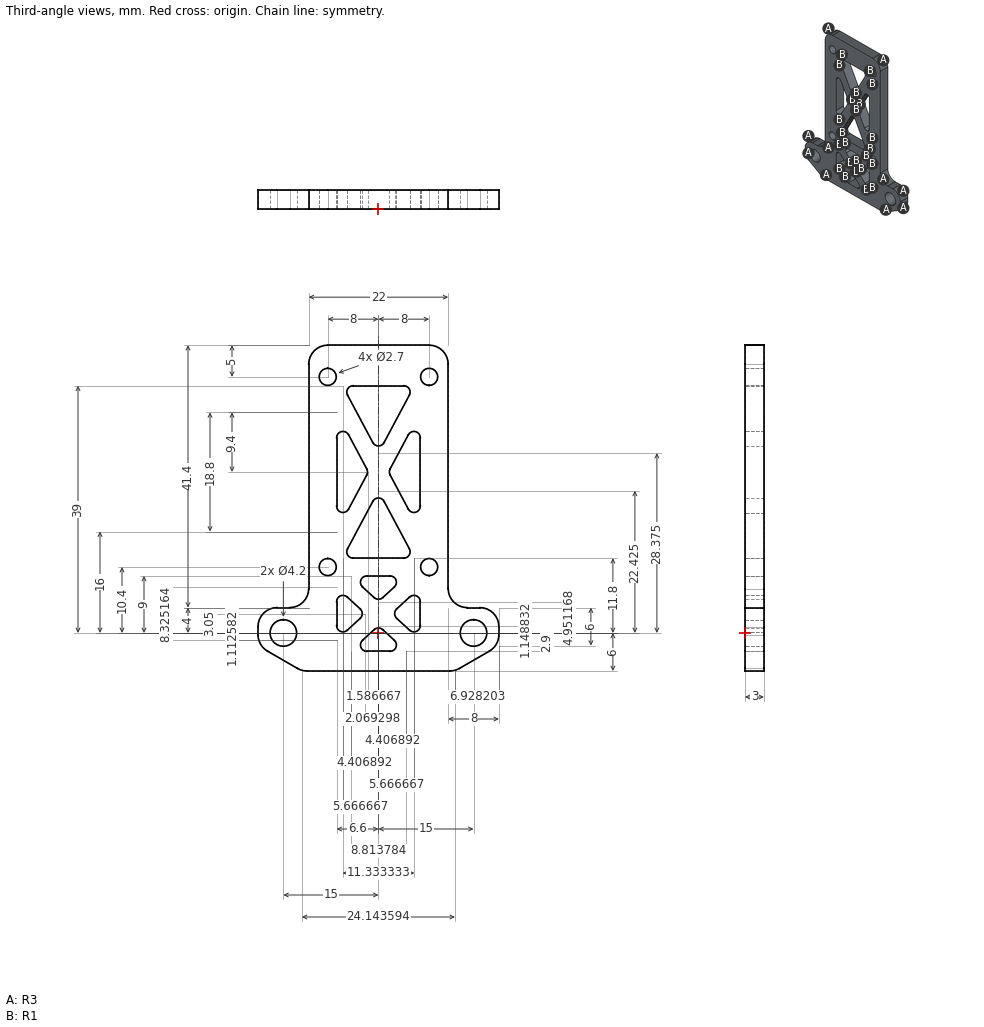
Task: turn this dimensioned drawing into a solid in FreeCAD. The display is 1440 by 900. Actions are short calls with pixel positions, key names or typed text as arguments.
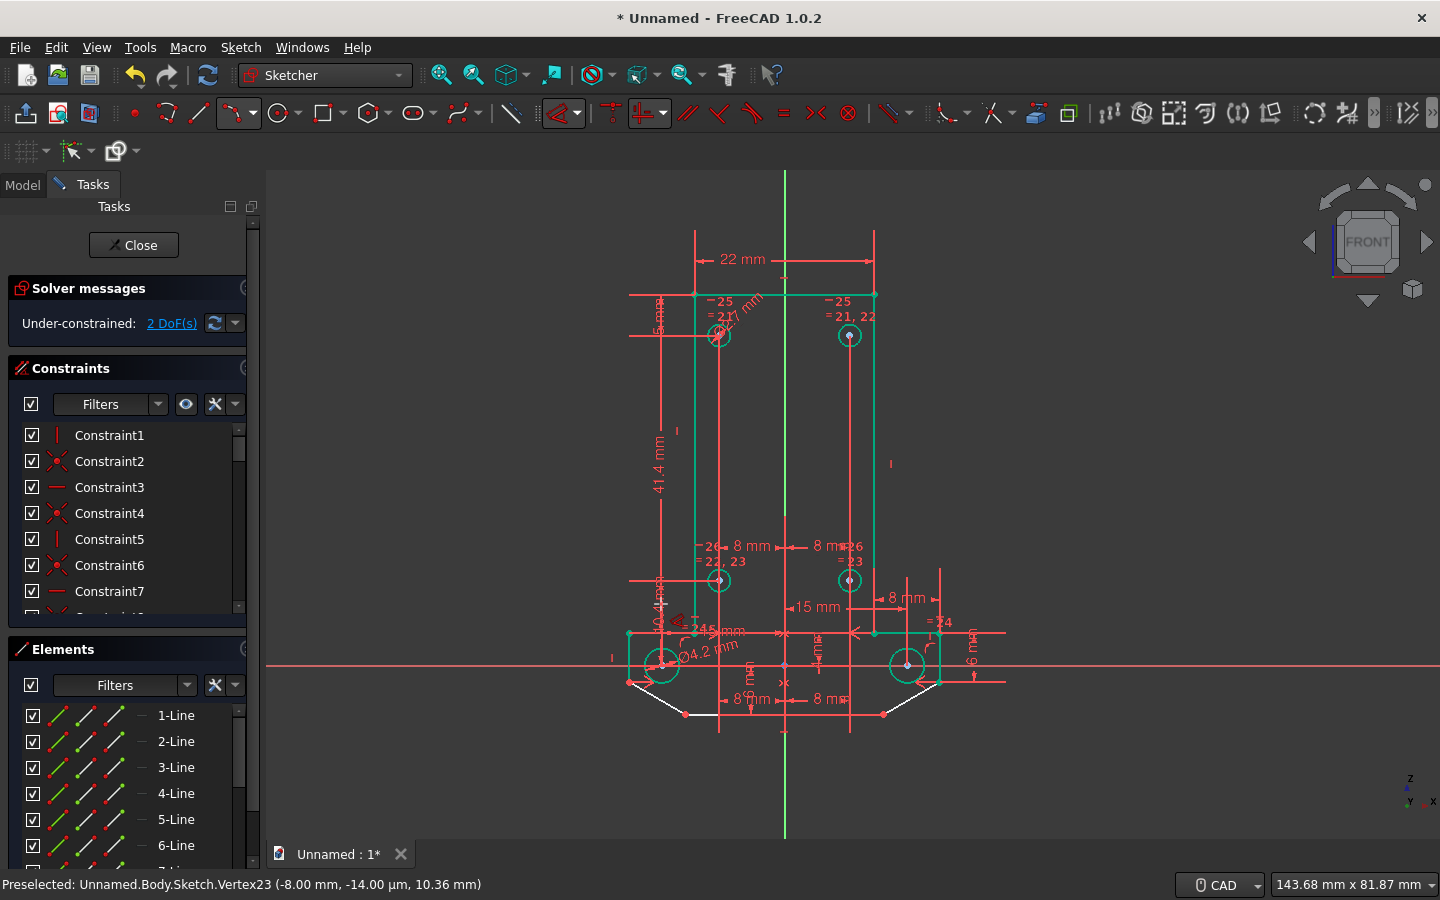
click(824, 715)
click(739, 749)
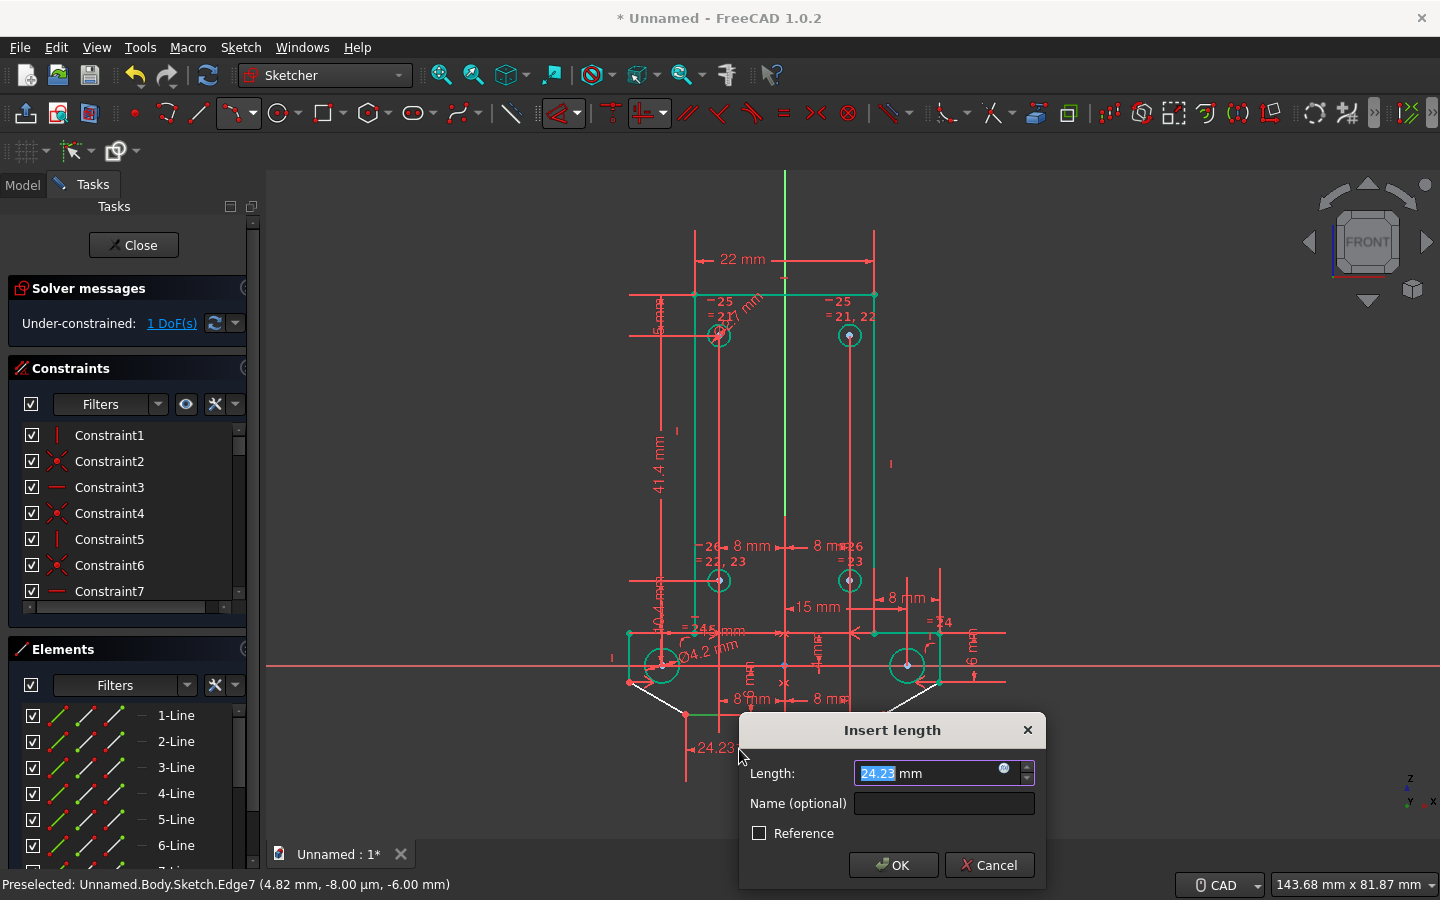
text(24.143594)
key(Return)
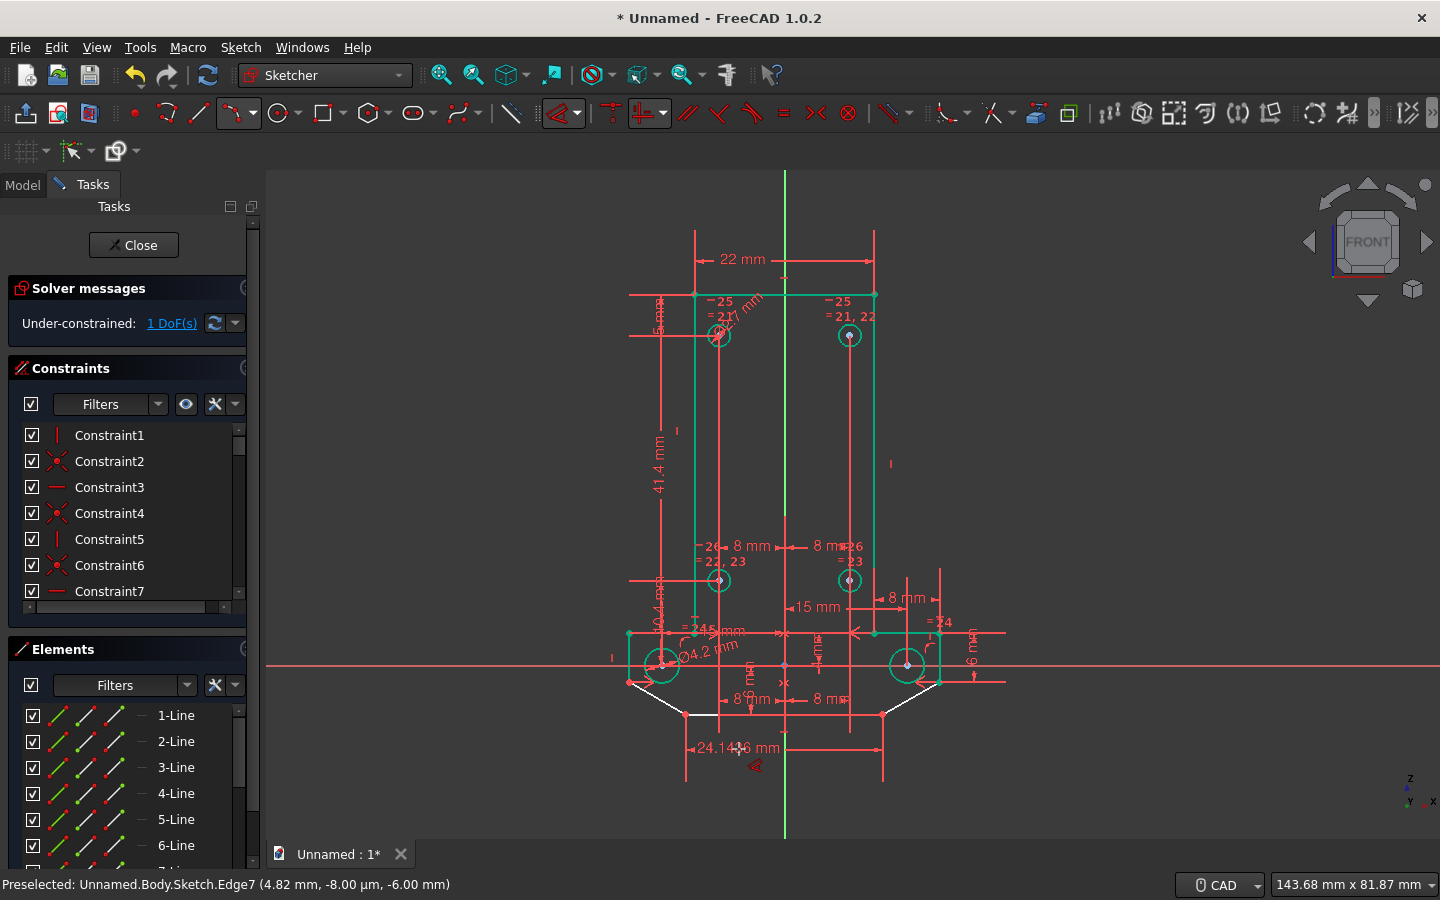
click(923, 692)
click(911, 749)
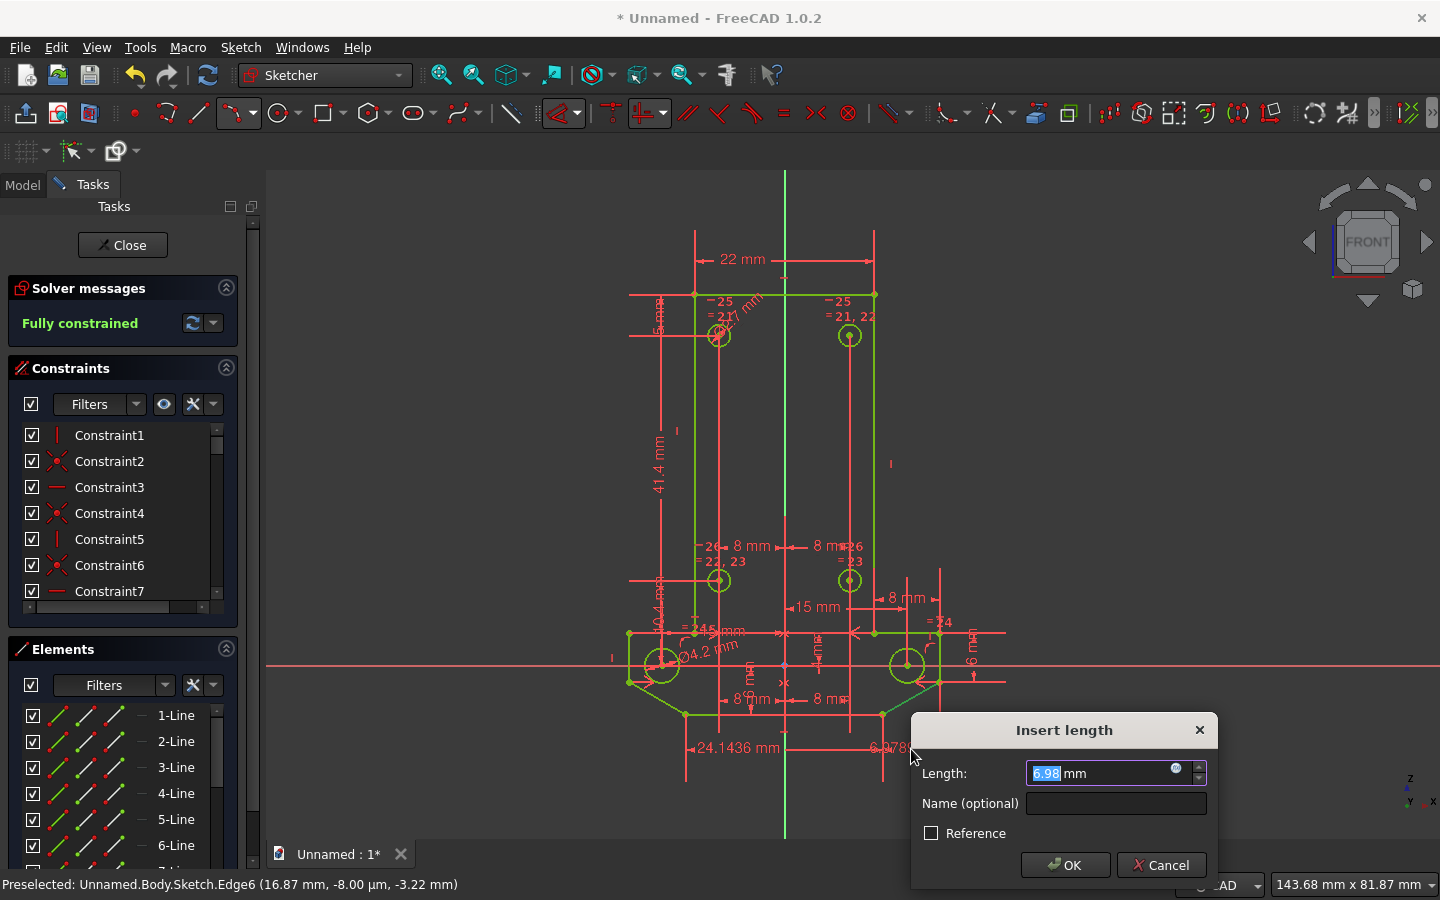
text(6.928203)
key(Return)
key(Escape)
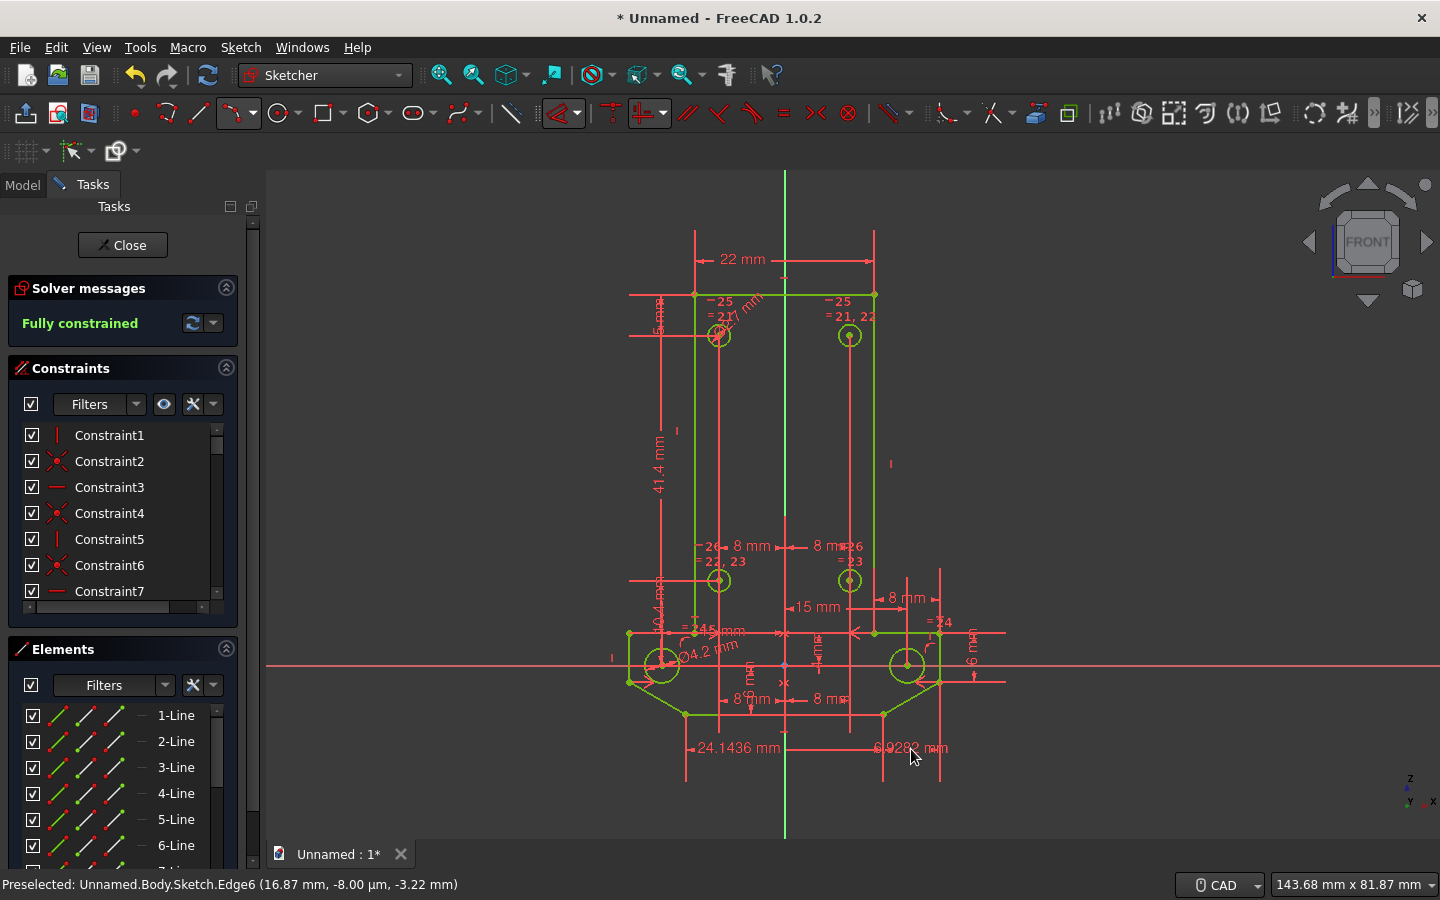
click(123, 245)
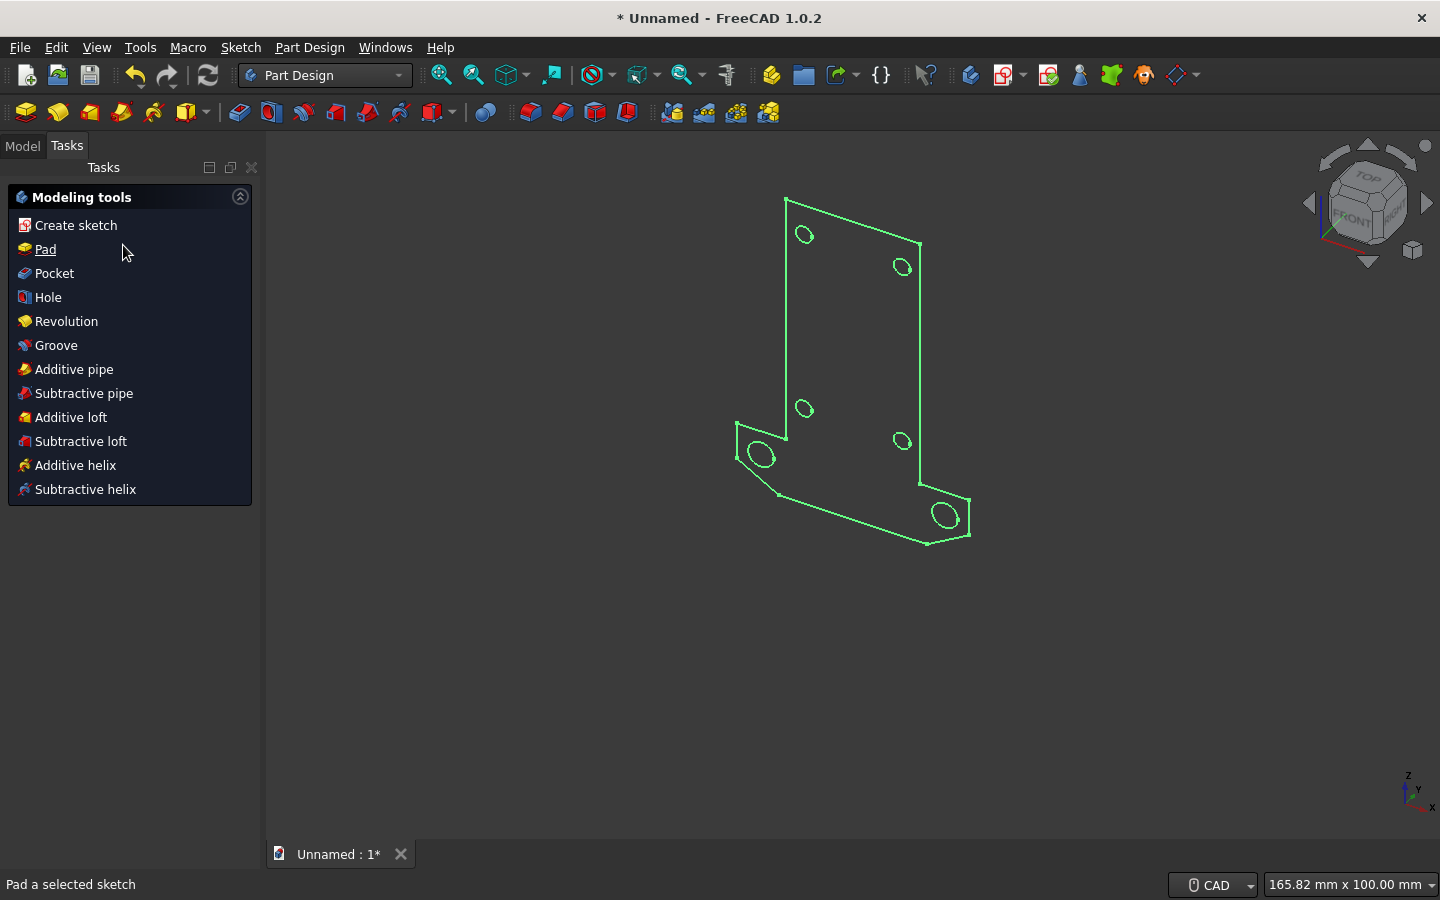
click(26, 112)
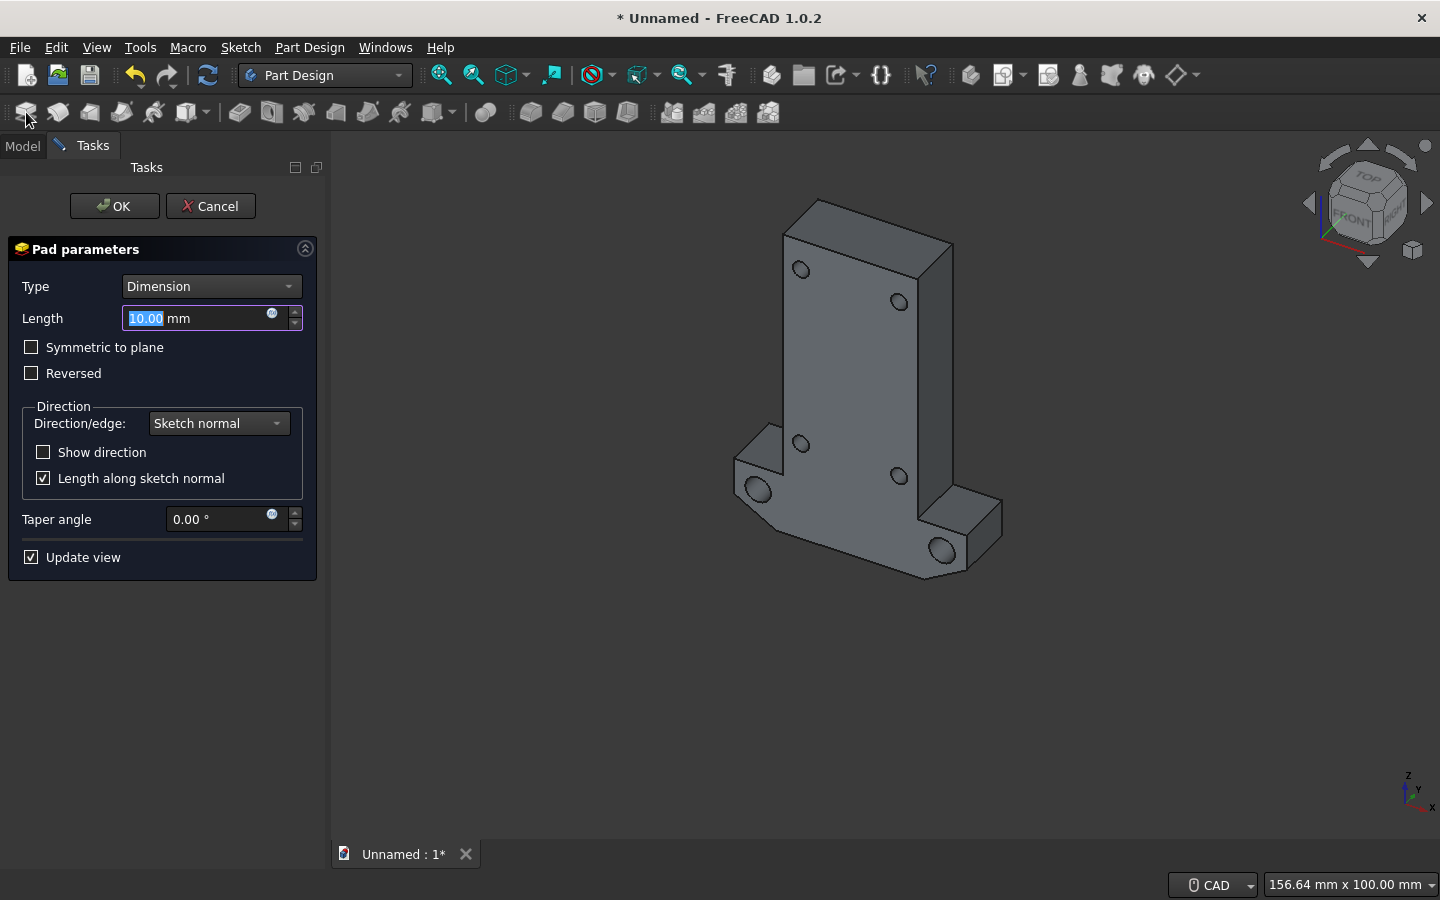
text(3)
key(Tab)